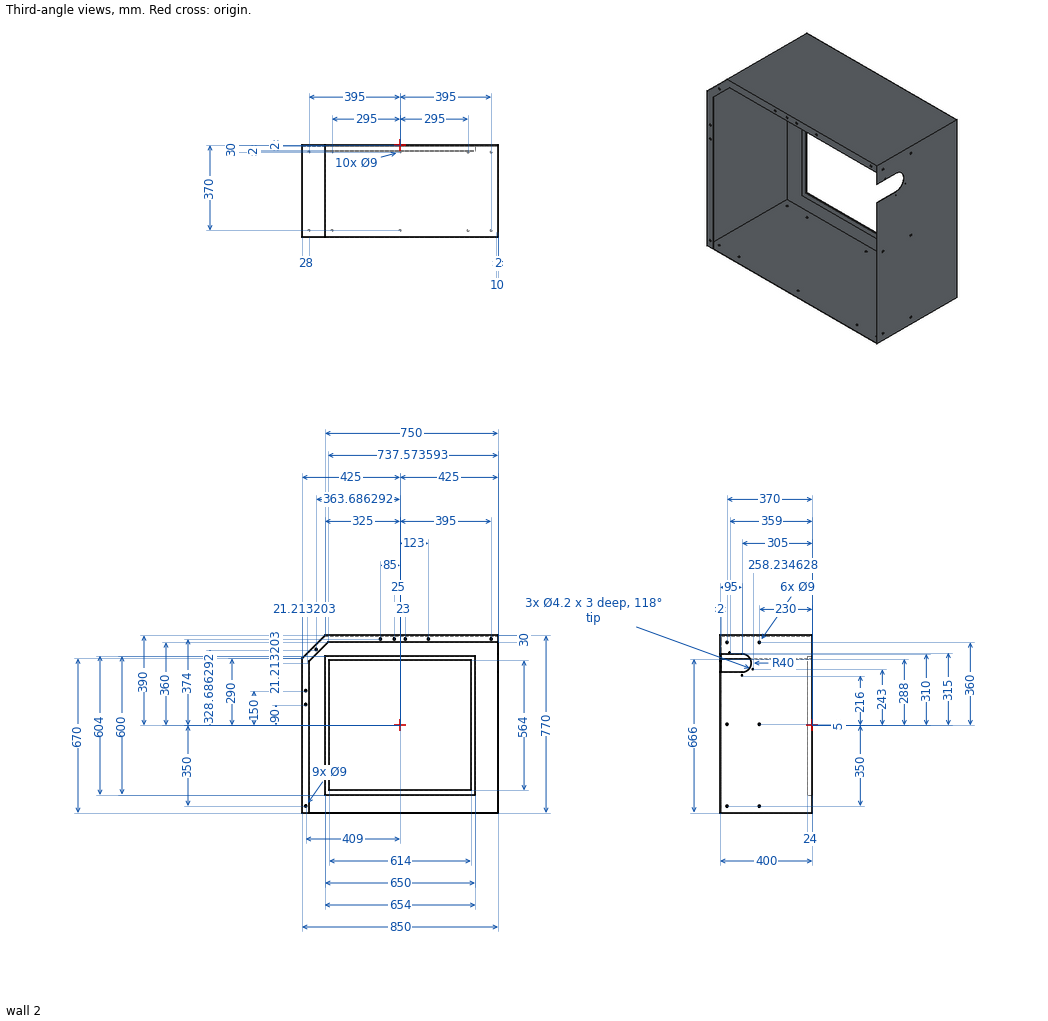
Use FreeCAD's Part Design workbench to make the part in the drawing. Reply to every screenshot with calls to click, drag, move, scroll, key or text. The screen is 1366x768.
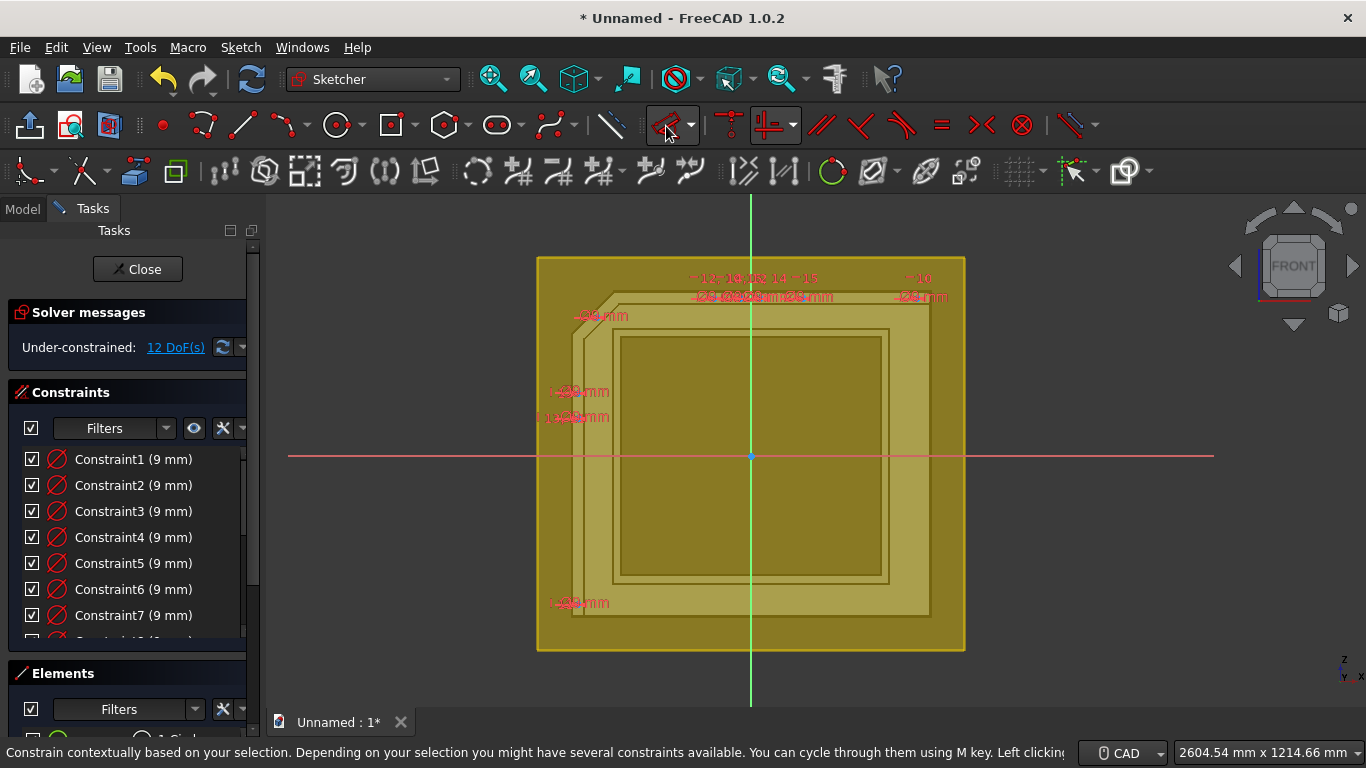
click(715, 299)
click(733, 265)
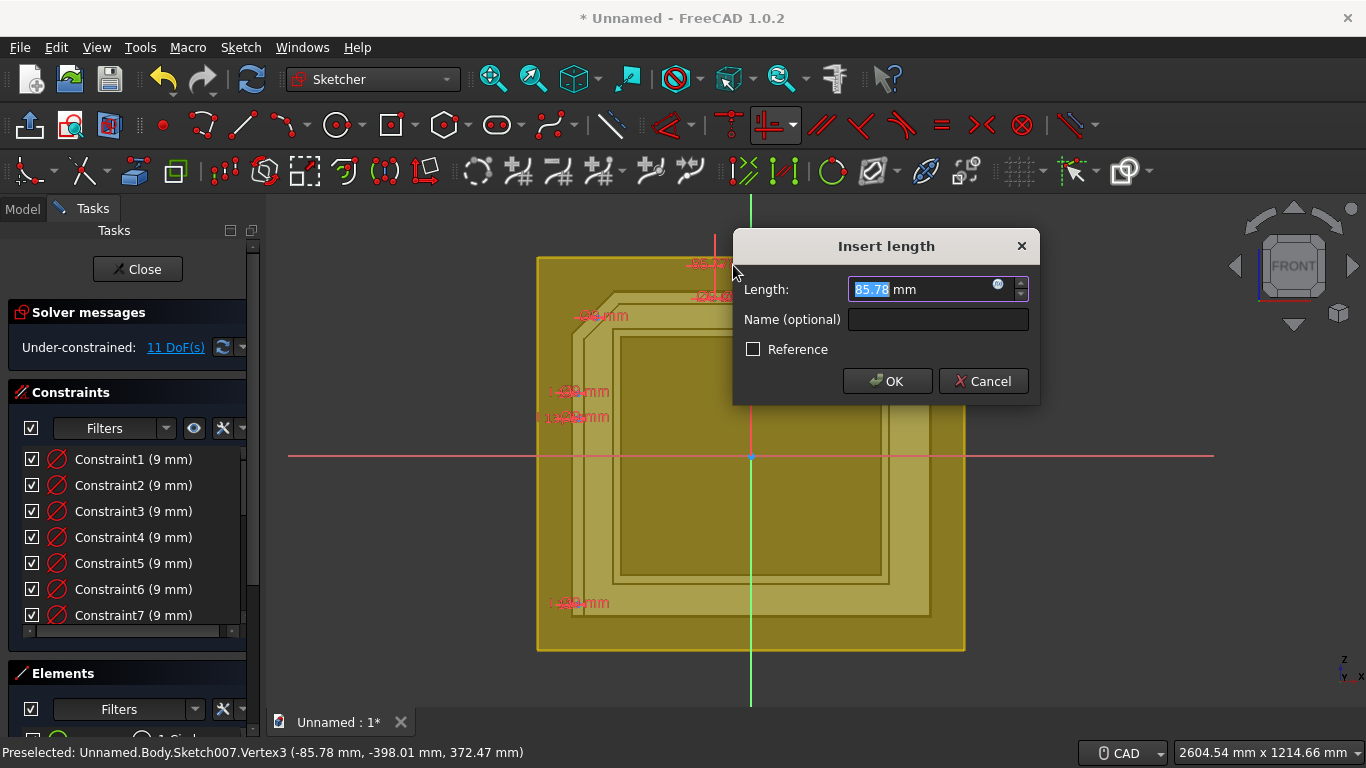
text(85)
key(Return)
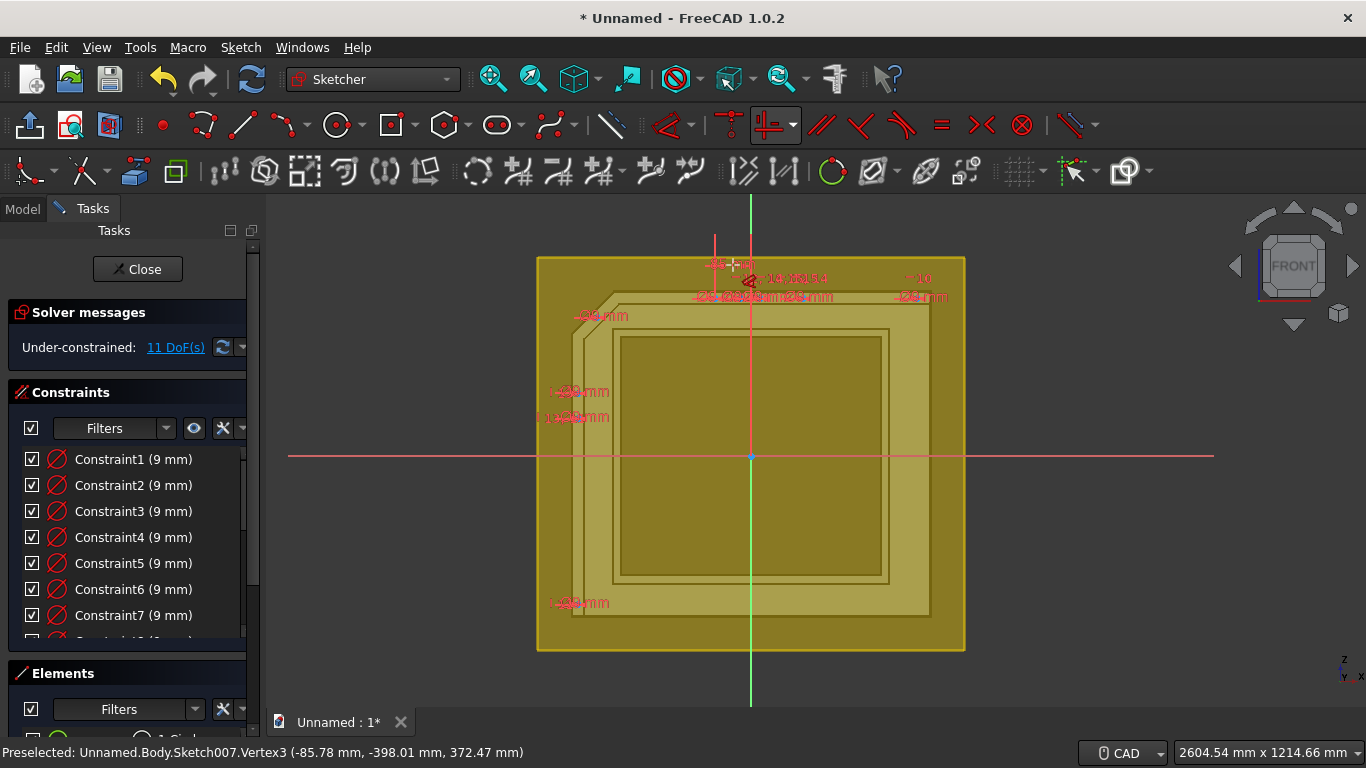
click(579, 419)
click(545, 437)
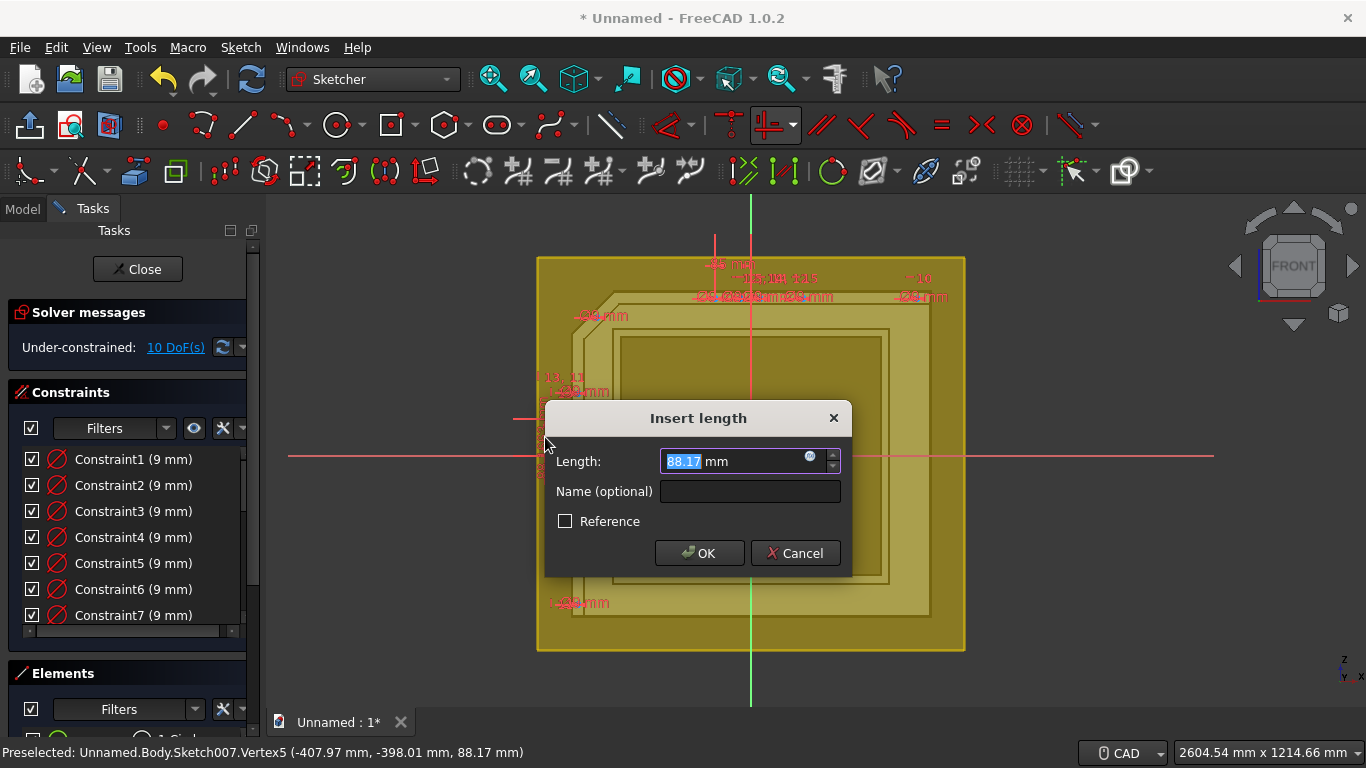
text(90)
key(Return)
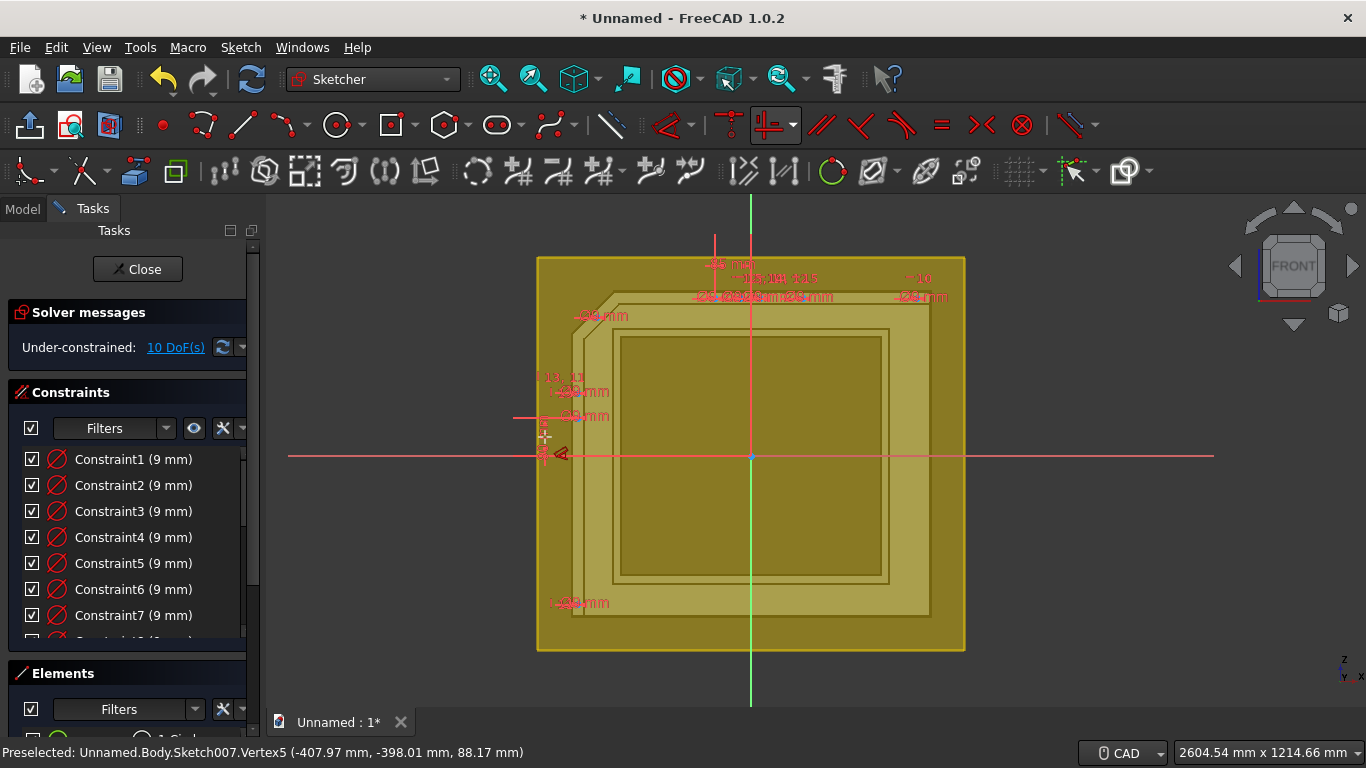
scroll(740, 299, up, 7)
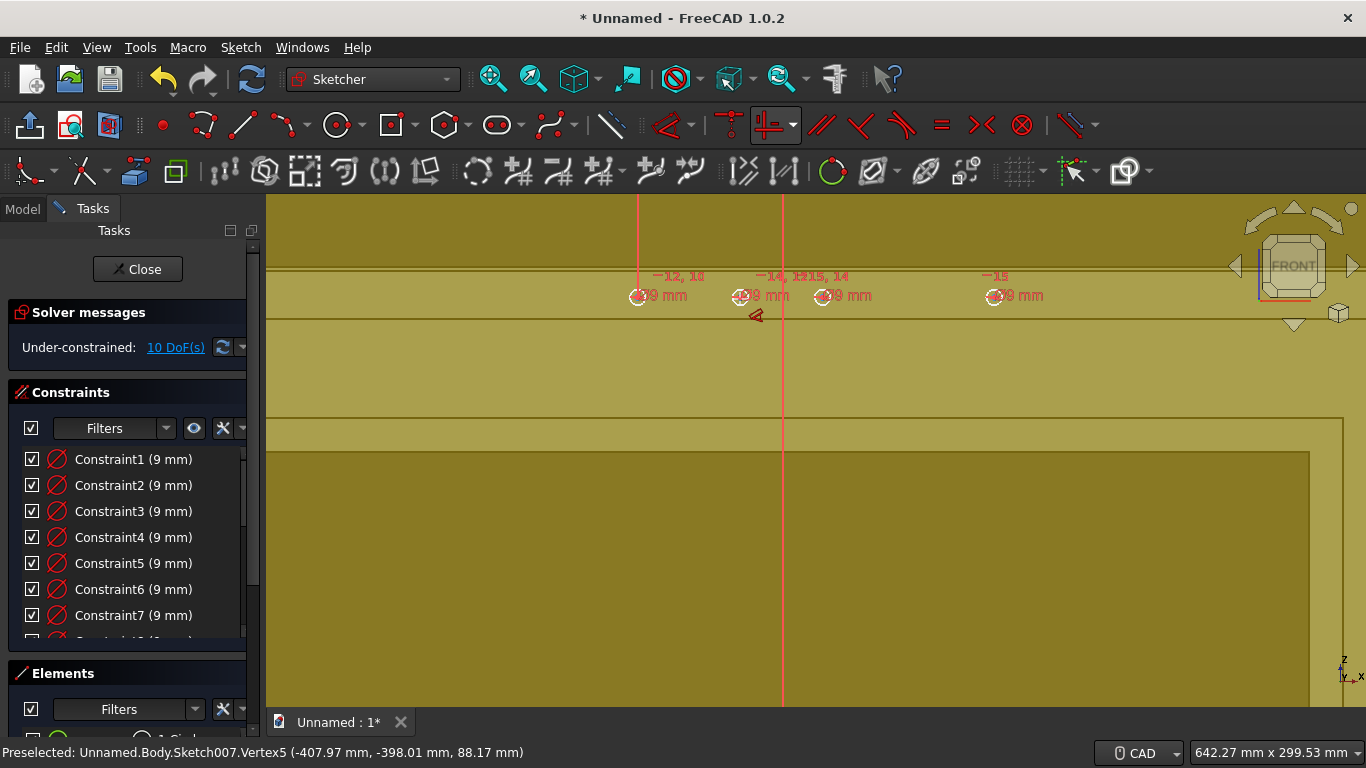
click(740, 297)
click(762, 263)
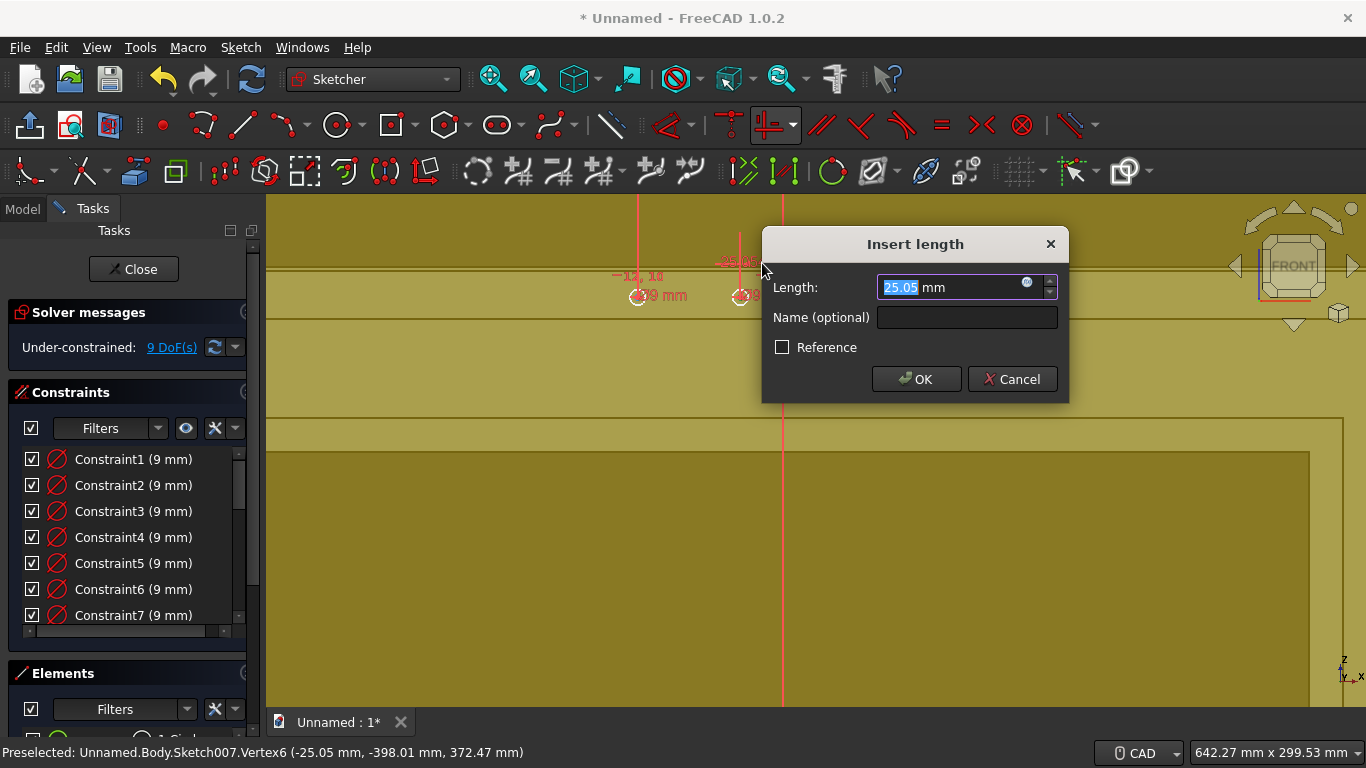
text(25)
key(Return)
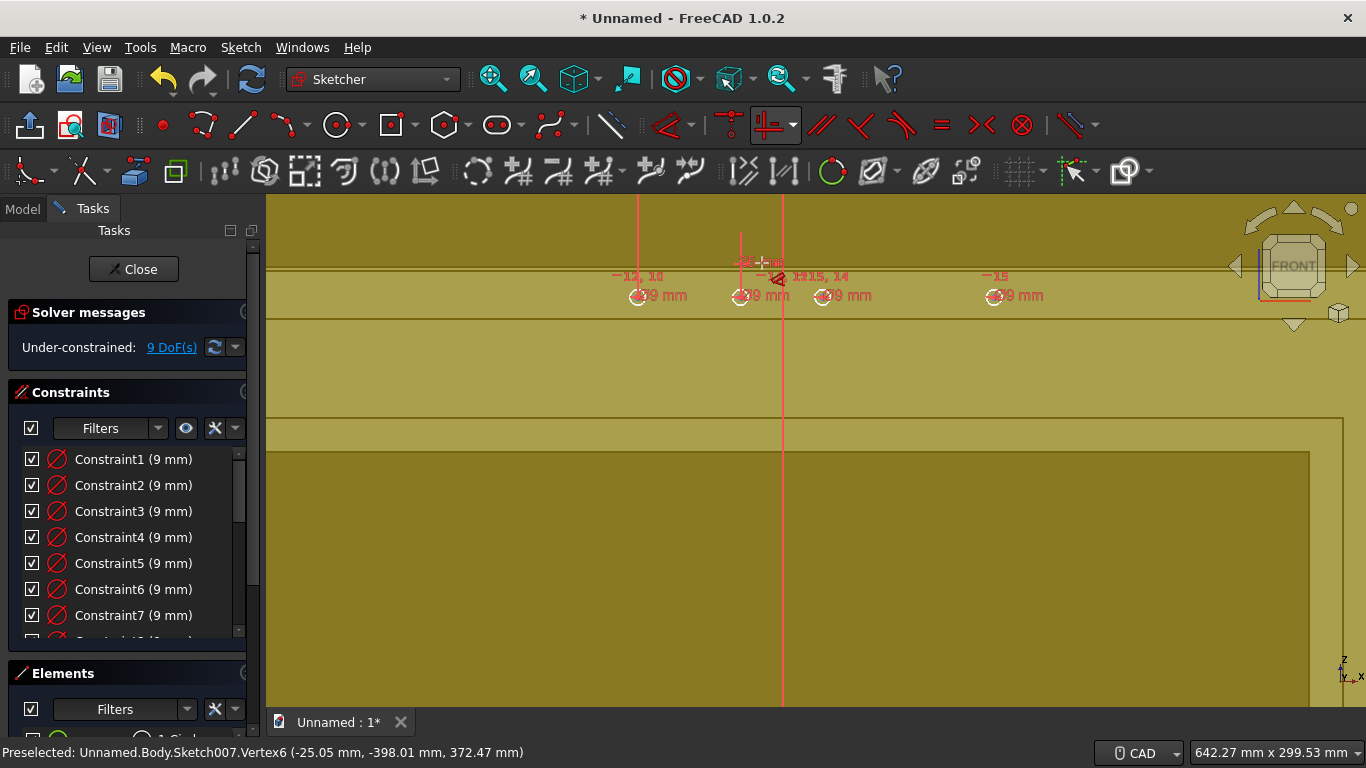
click(823, 297)
click(803, 239)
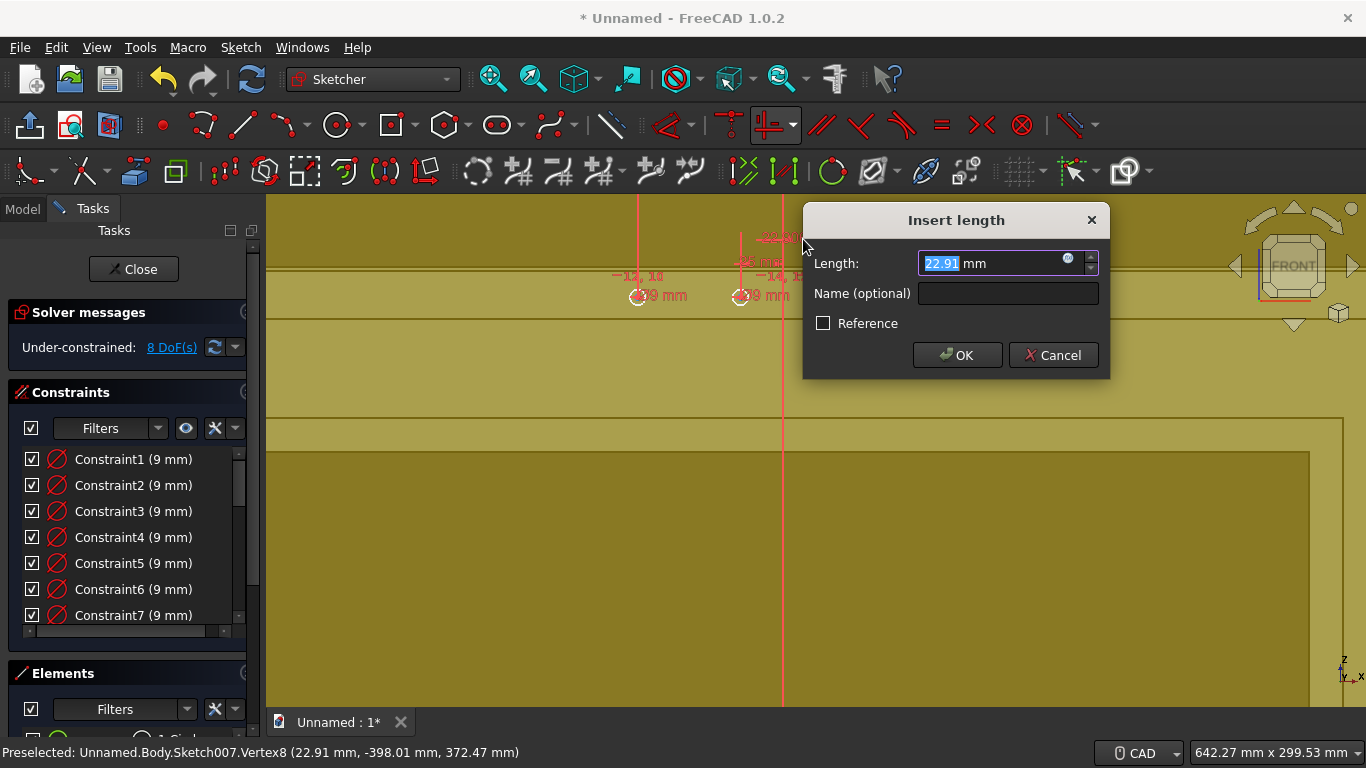
text(23)
key(Return)